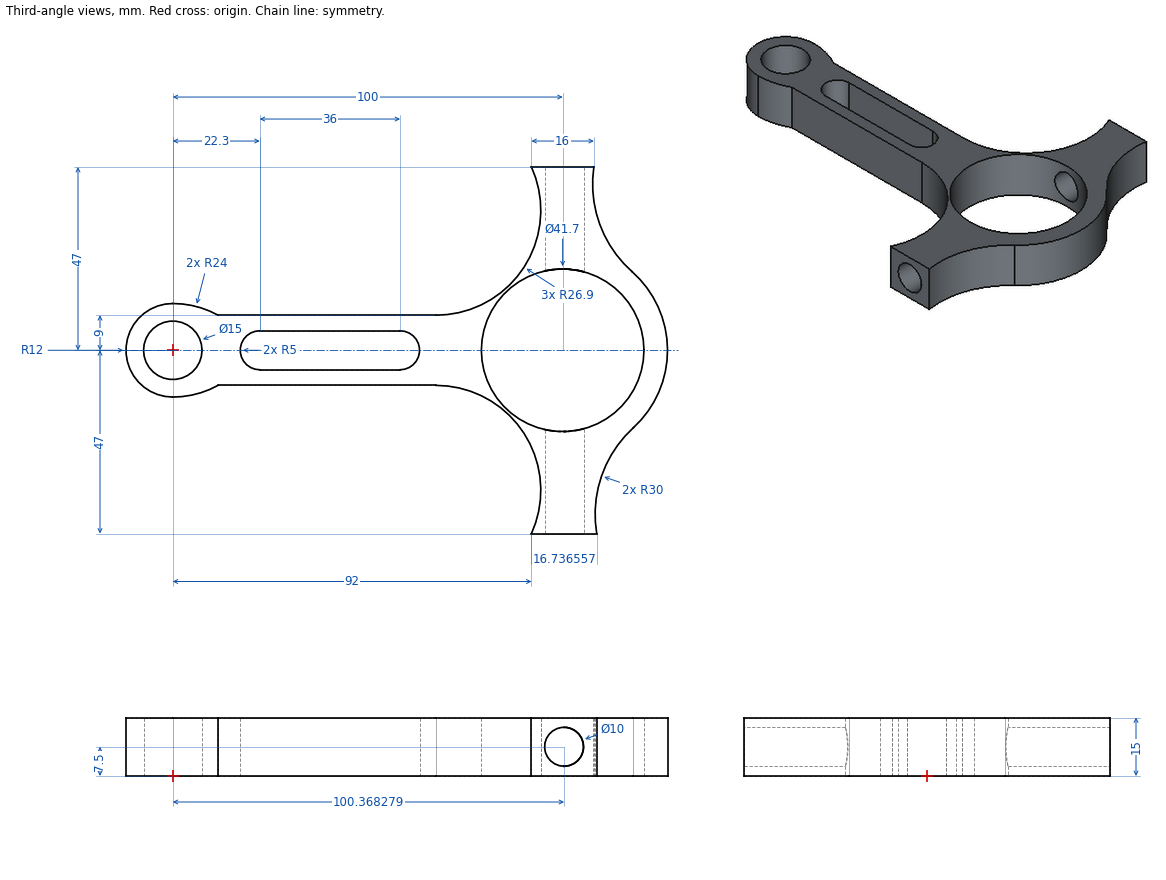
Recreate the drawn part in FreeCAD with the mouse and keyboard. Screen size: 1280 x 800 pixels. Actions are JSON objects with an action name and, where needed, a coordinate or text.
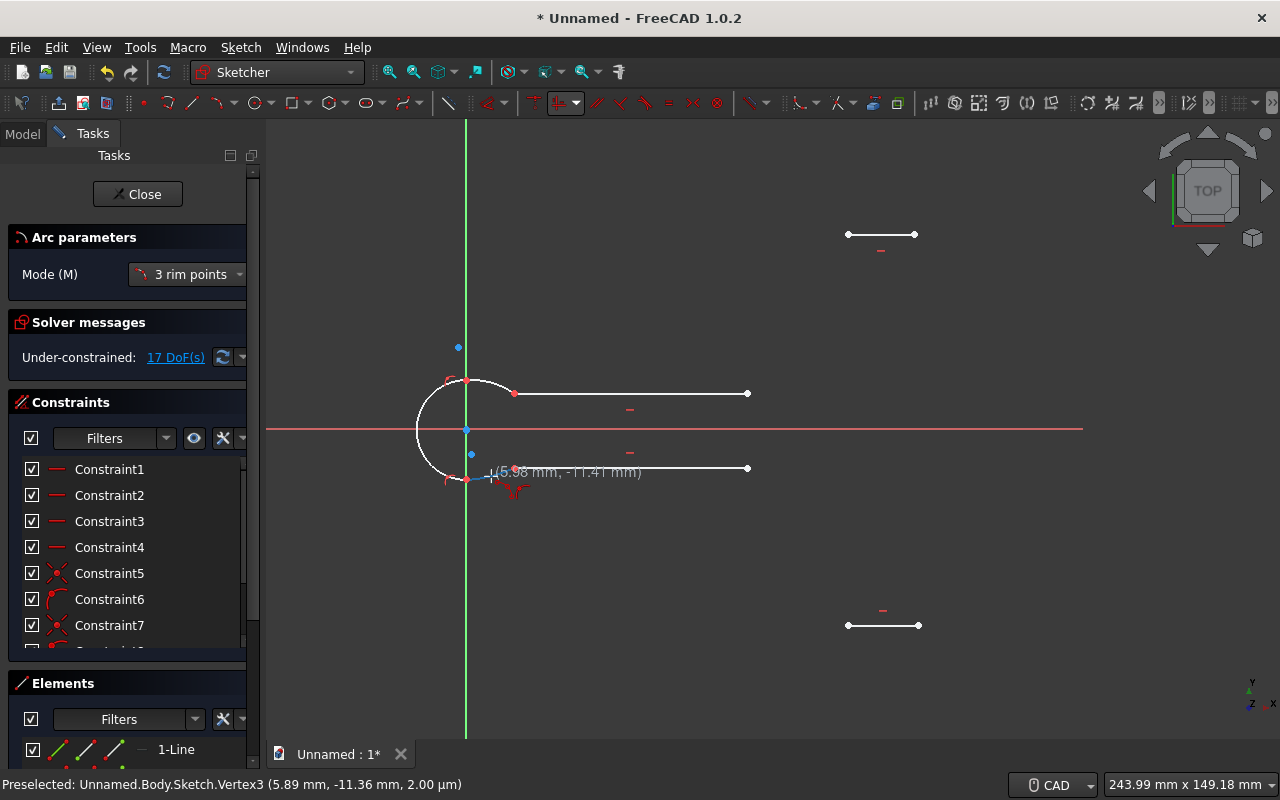
{"action": "left_click", "coordinate": [747, 468]}
{"action": "left_click", "coordinate": [849, 626]}
{"action": "left_click", "coordinate": [841, 518]}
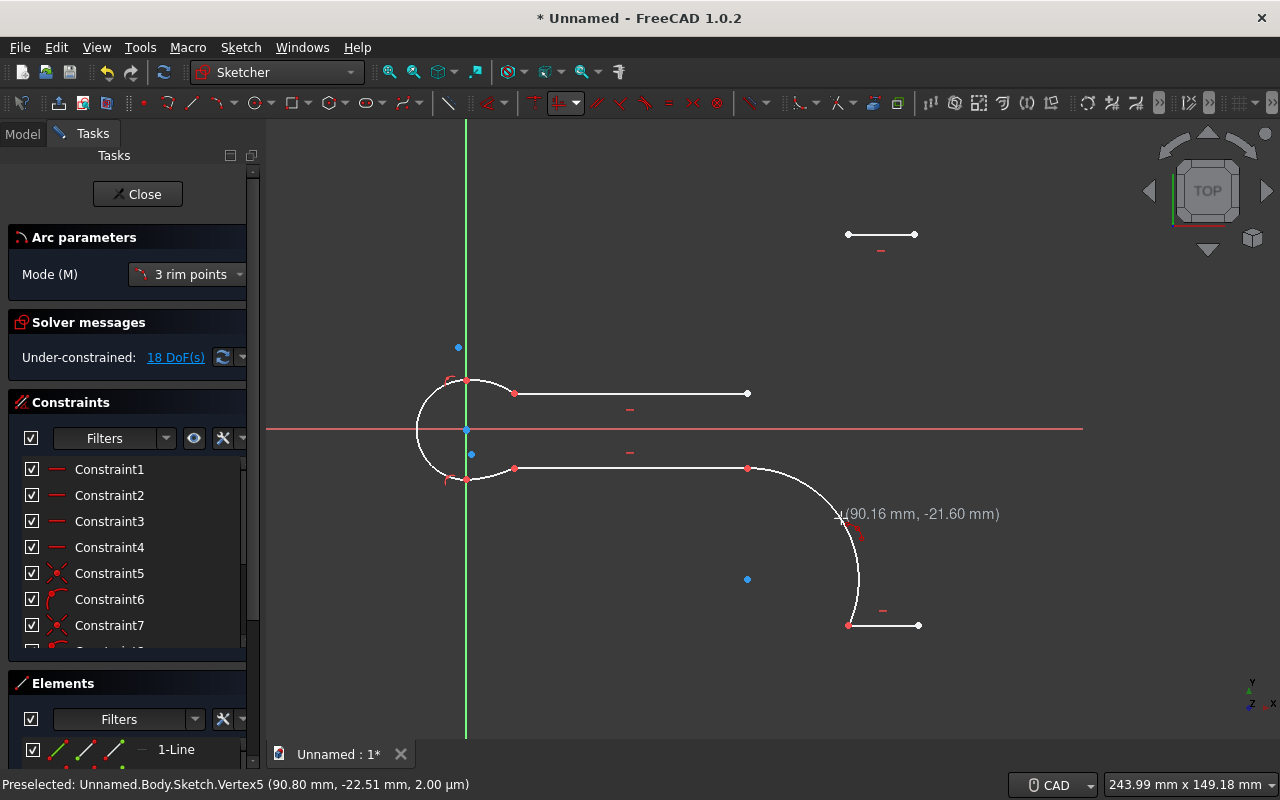
{"action": "left_click", "coordinate": [918, 626]}
{"action": "left_click", "coordinate": [957, 512]}
{"action": "left_click", "coordinate": [923, 563]}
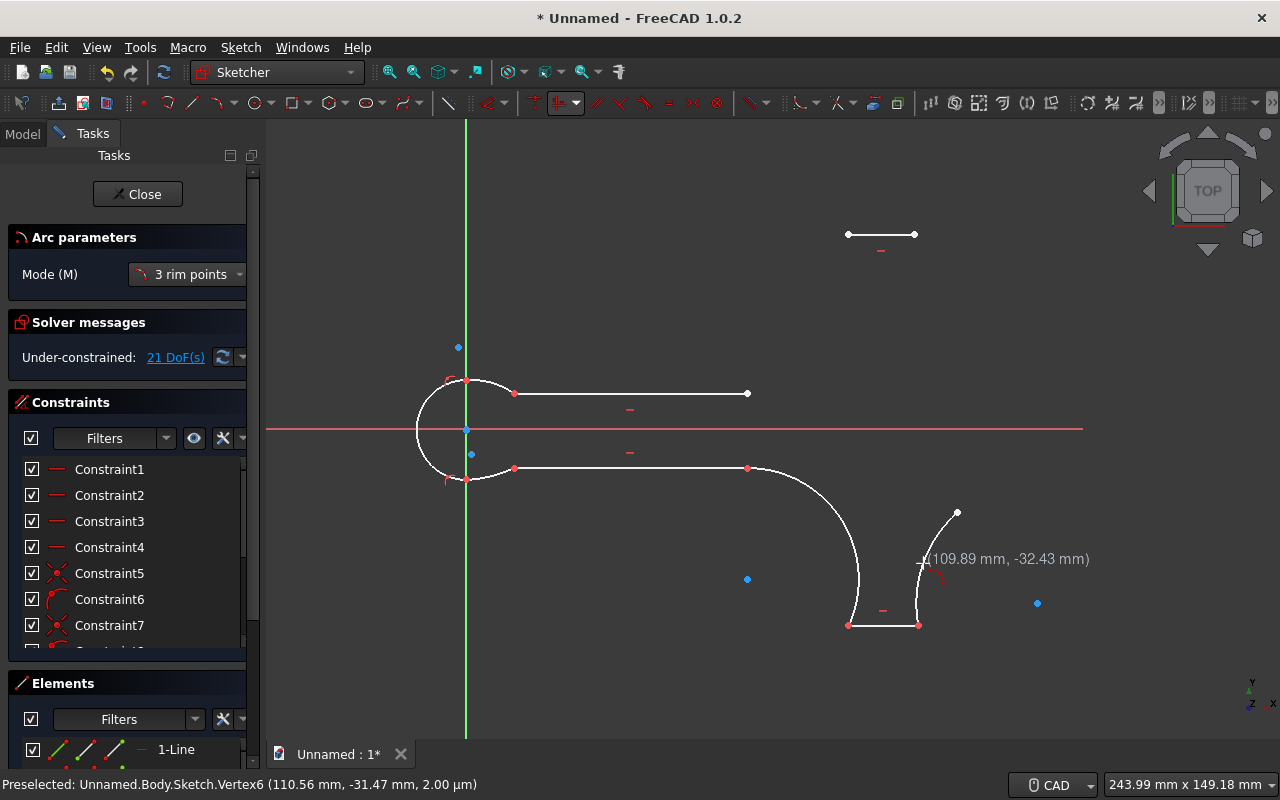
{"action": "left_click", "coordinate": [957, 513]}
{"action": "left_click", "coordinate": [956, 345]}
{"action": "left_click", "coordinate": [992, 447]}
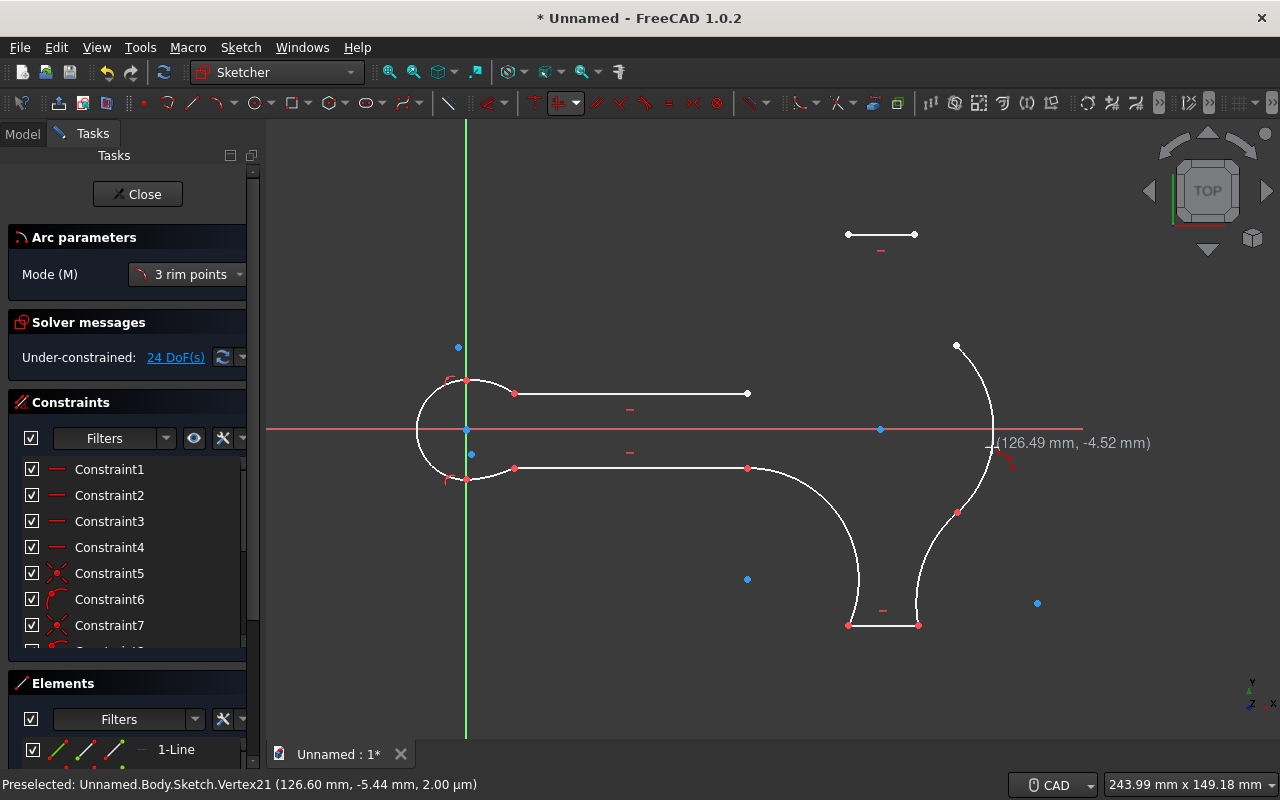
{"action": "left_click", "coordinate": [956, 346]}
{"action": "left_click", "coordinate": [915, 235]}
{"action": "left_click", "coordinate": [921, 295]}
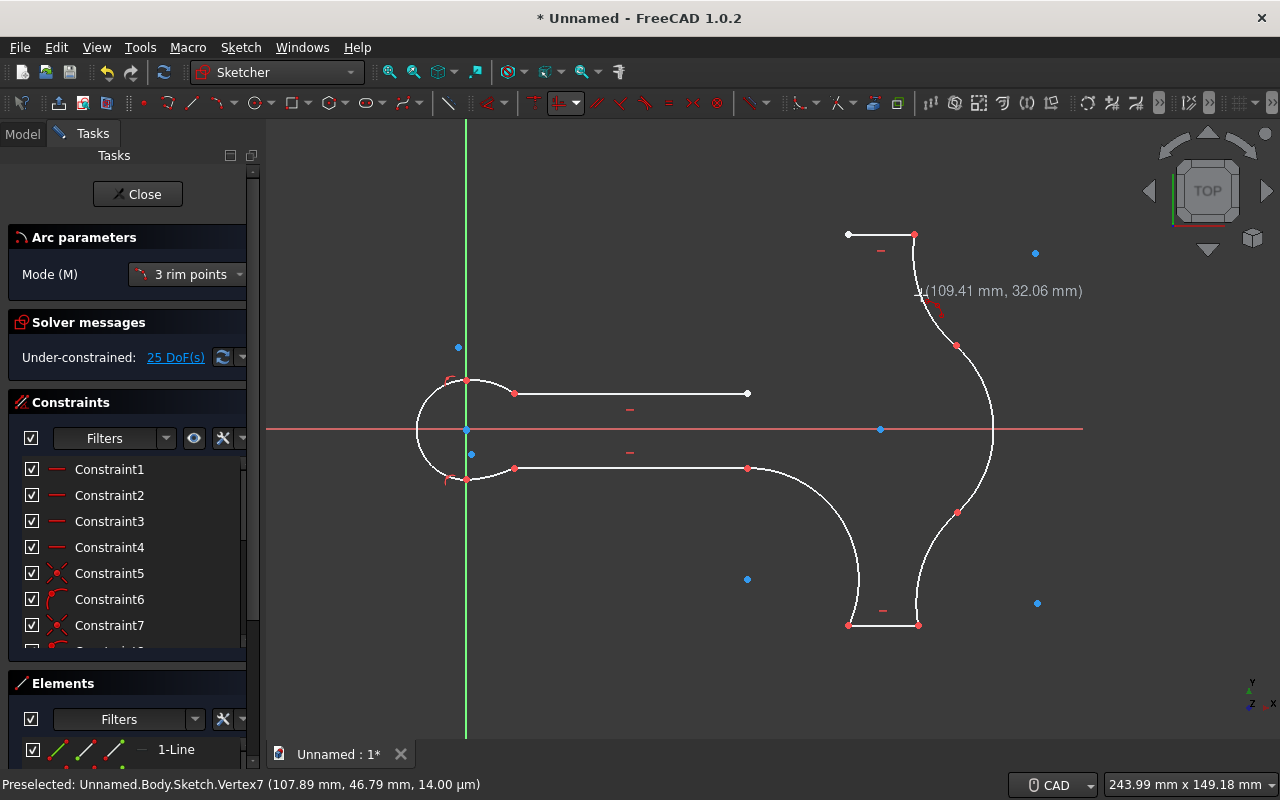
{"action": "left_click", "coordinate": [849, 235]}
{"action": "left_click", "coordinate": [747, 394]}
{"action": "left_click", "coordinate": [841, 341]}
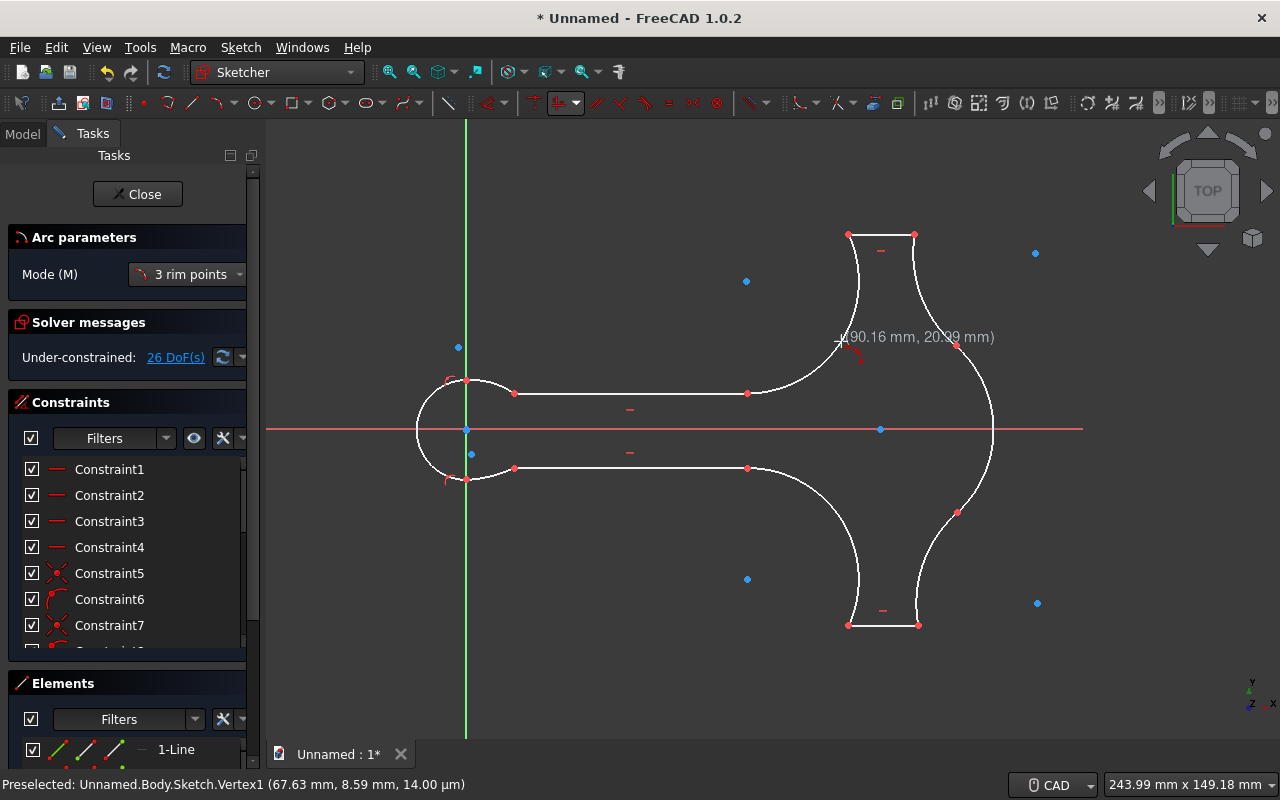
{"action": "left_click", "coordinate": [366, 104]}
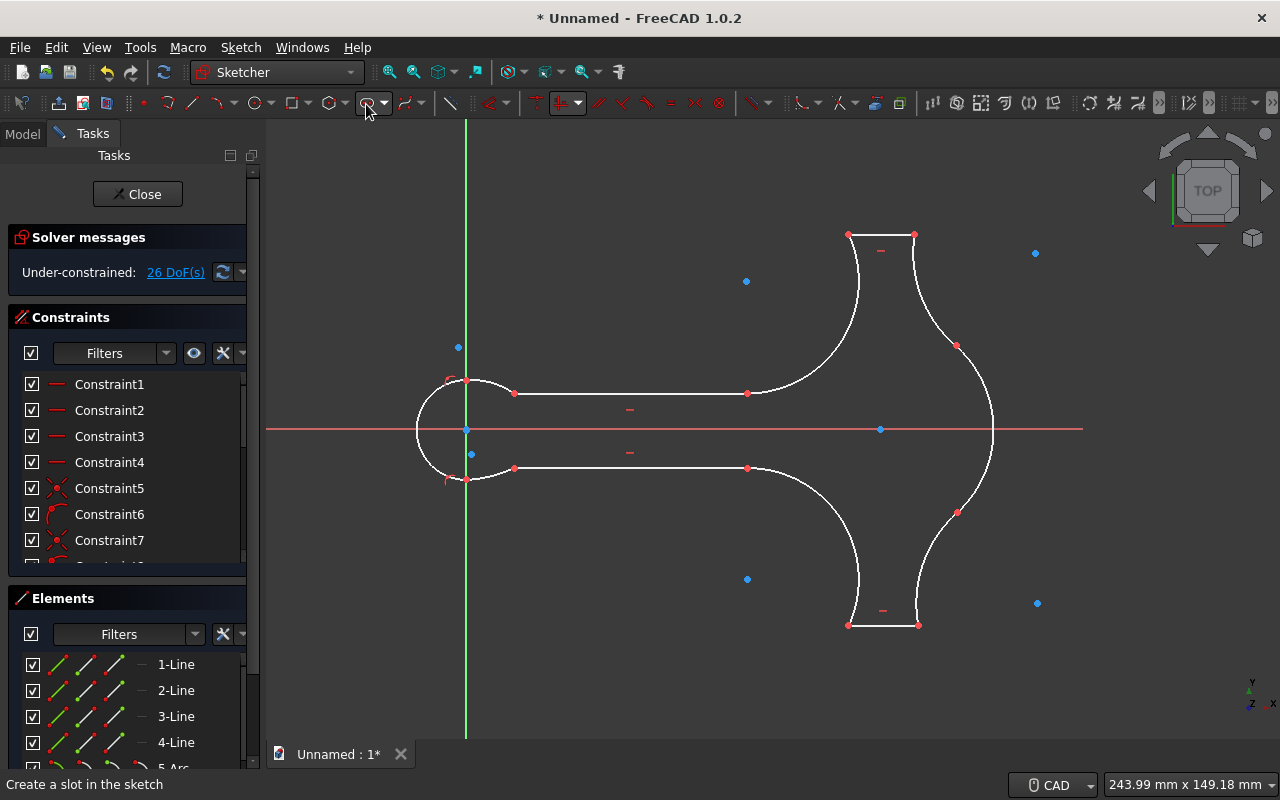
{"action": "left_click", "coordinate": [559, 429]}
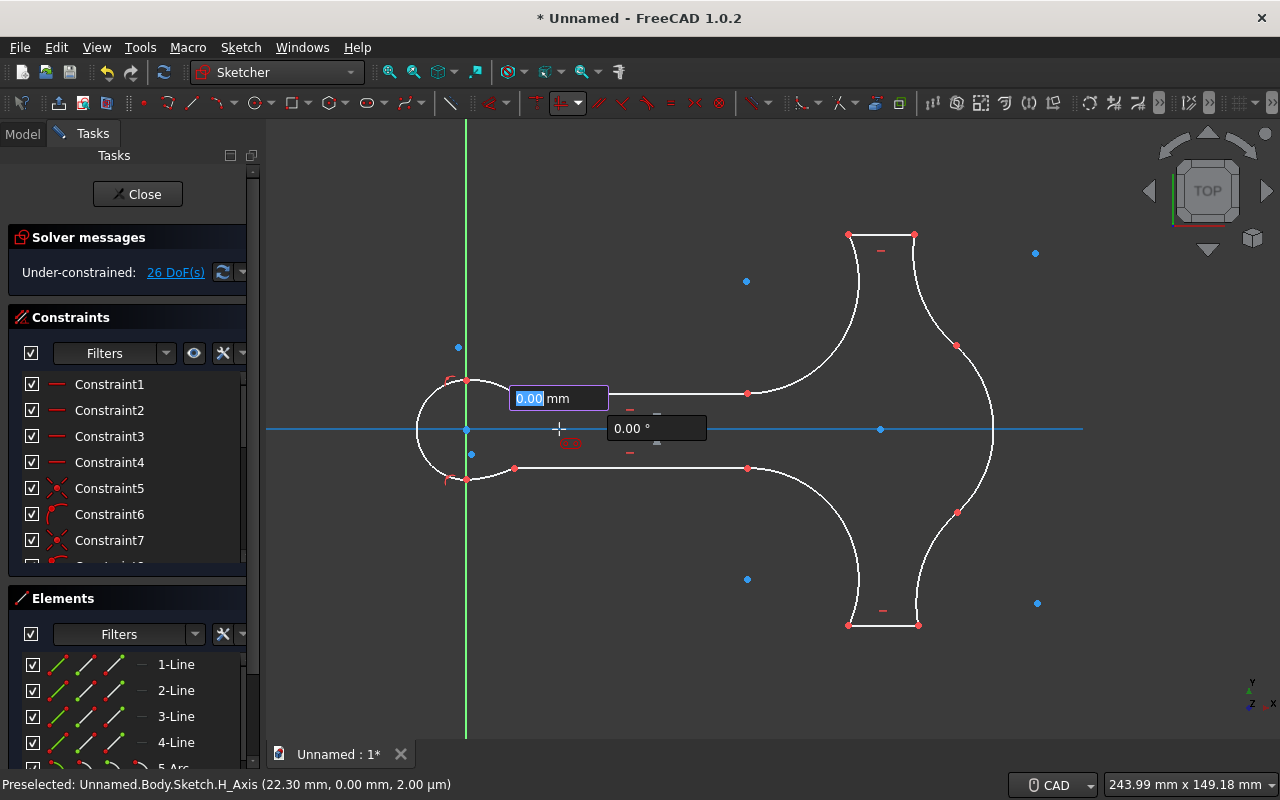
{"action": "left_click", "coordinate": [709, 420]}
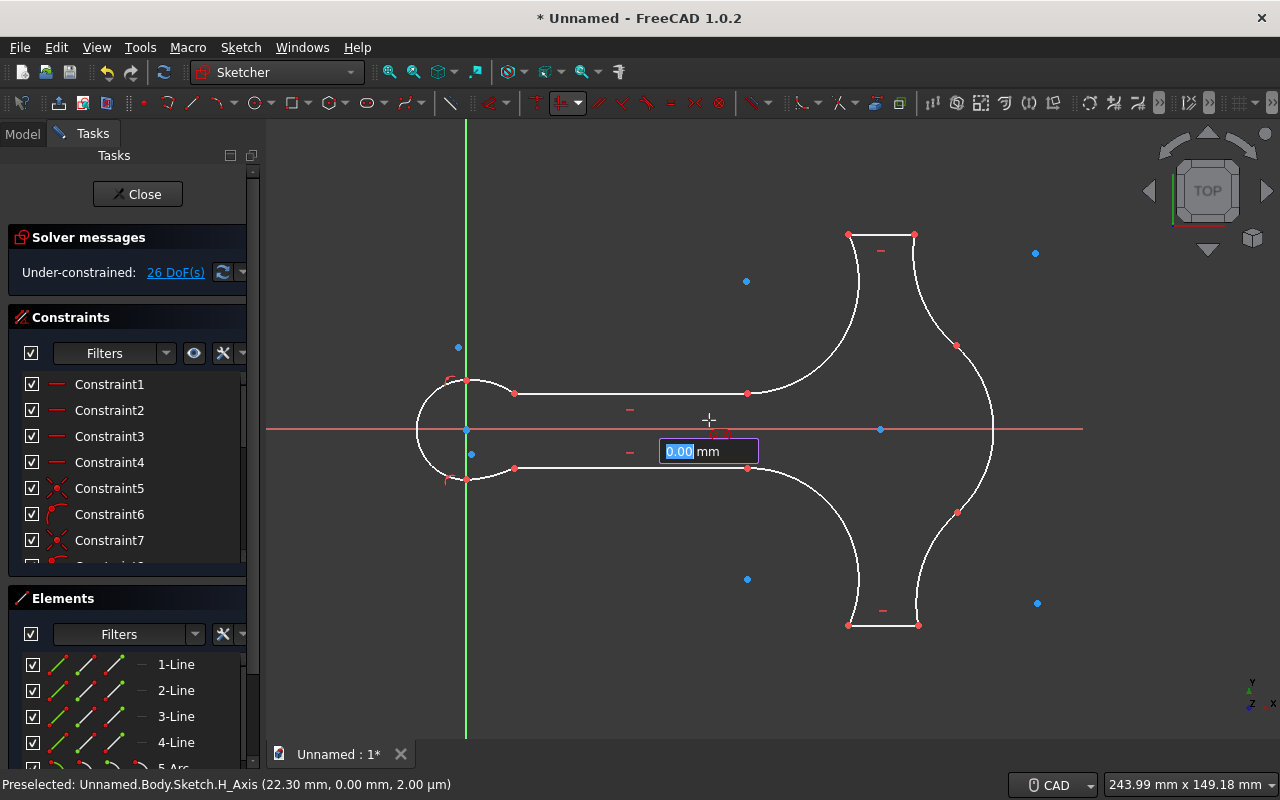
{"action": "left_click", "coordinate": [634, 450]}